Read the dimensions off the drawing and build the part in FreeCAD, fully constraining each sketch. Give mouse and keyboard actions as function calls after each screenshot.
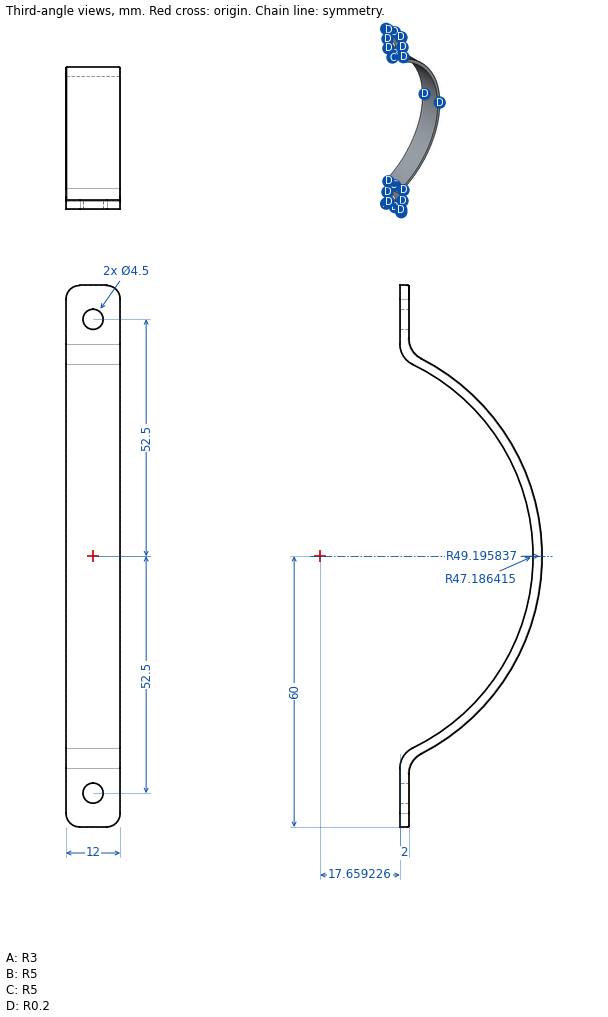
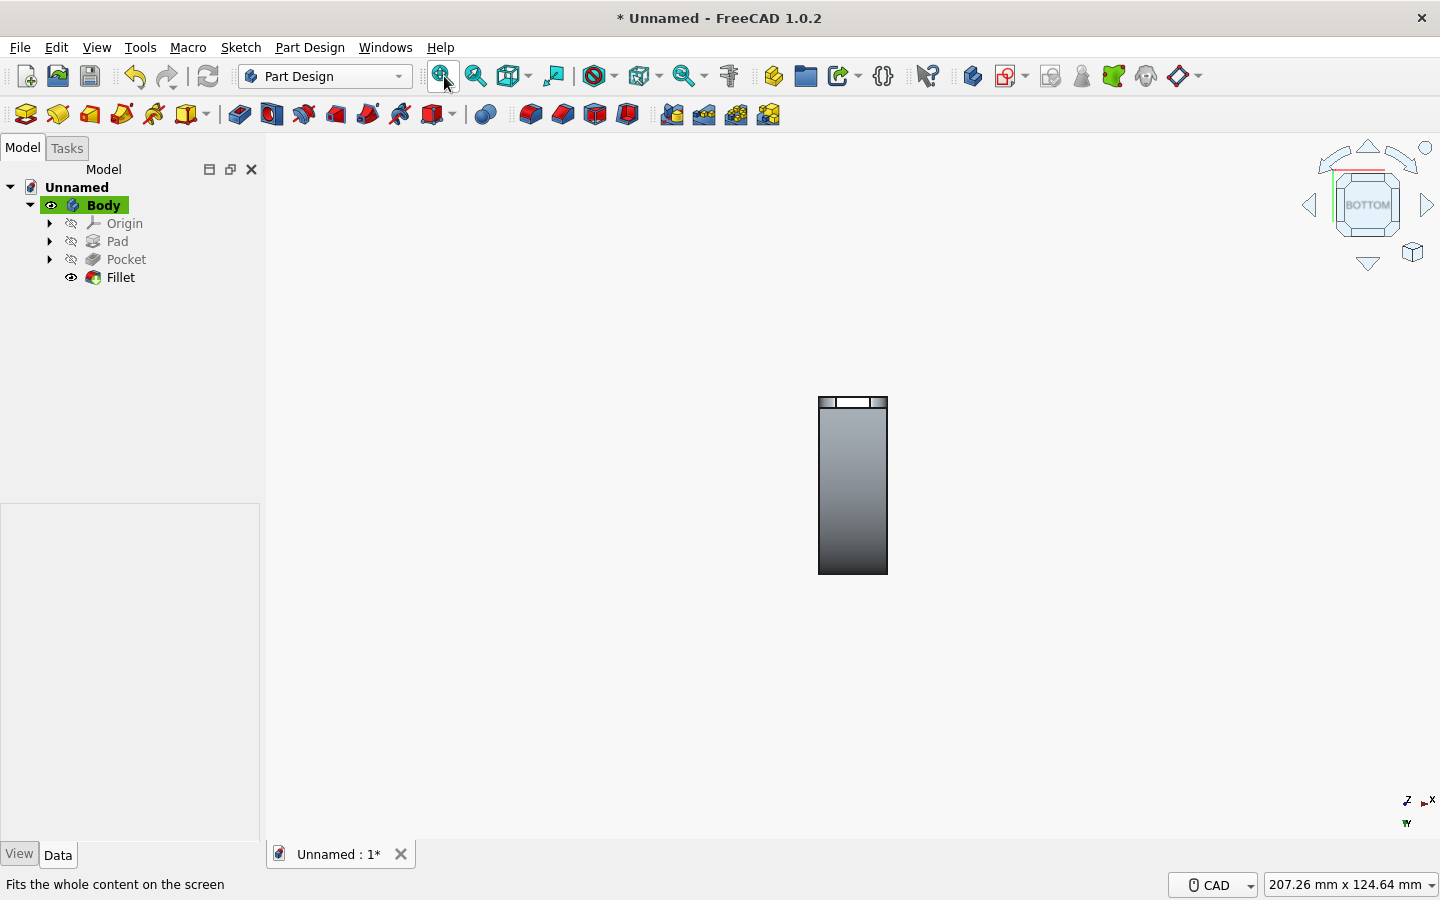
key(4)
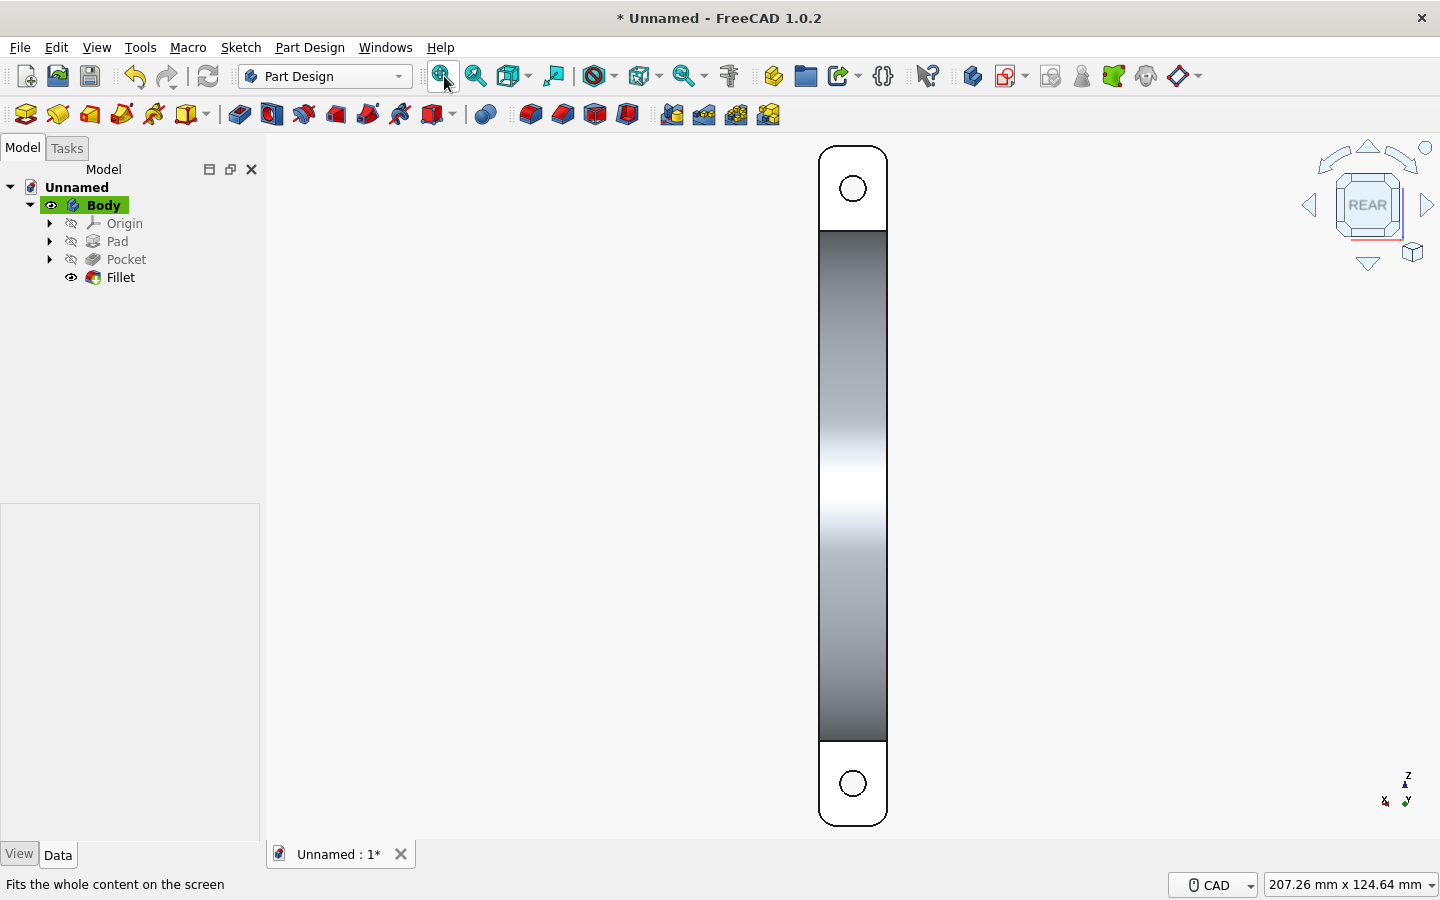
key(6)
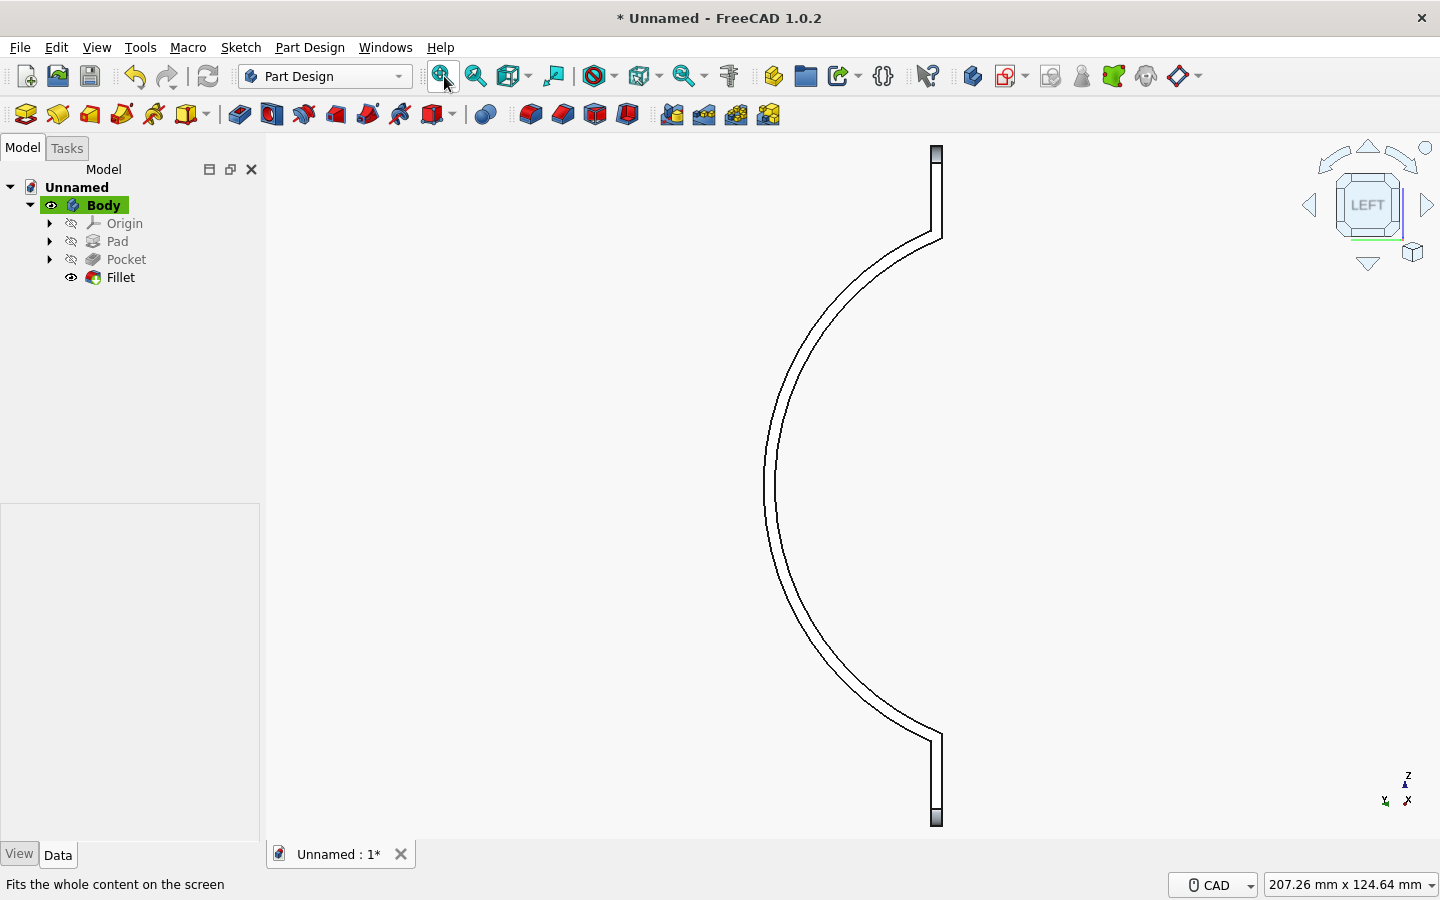
key(v)
key(3)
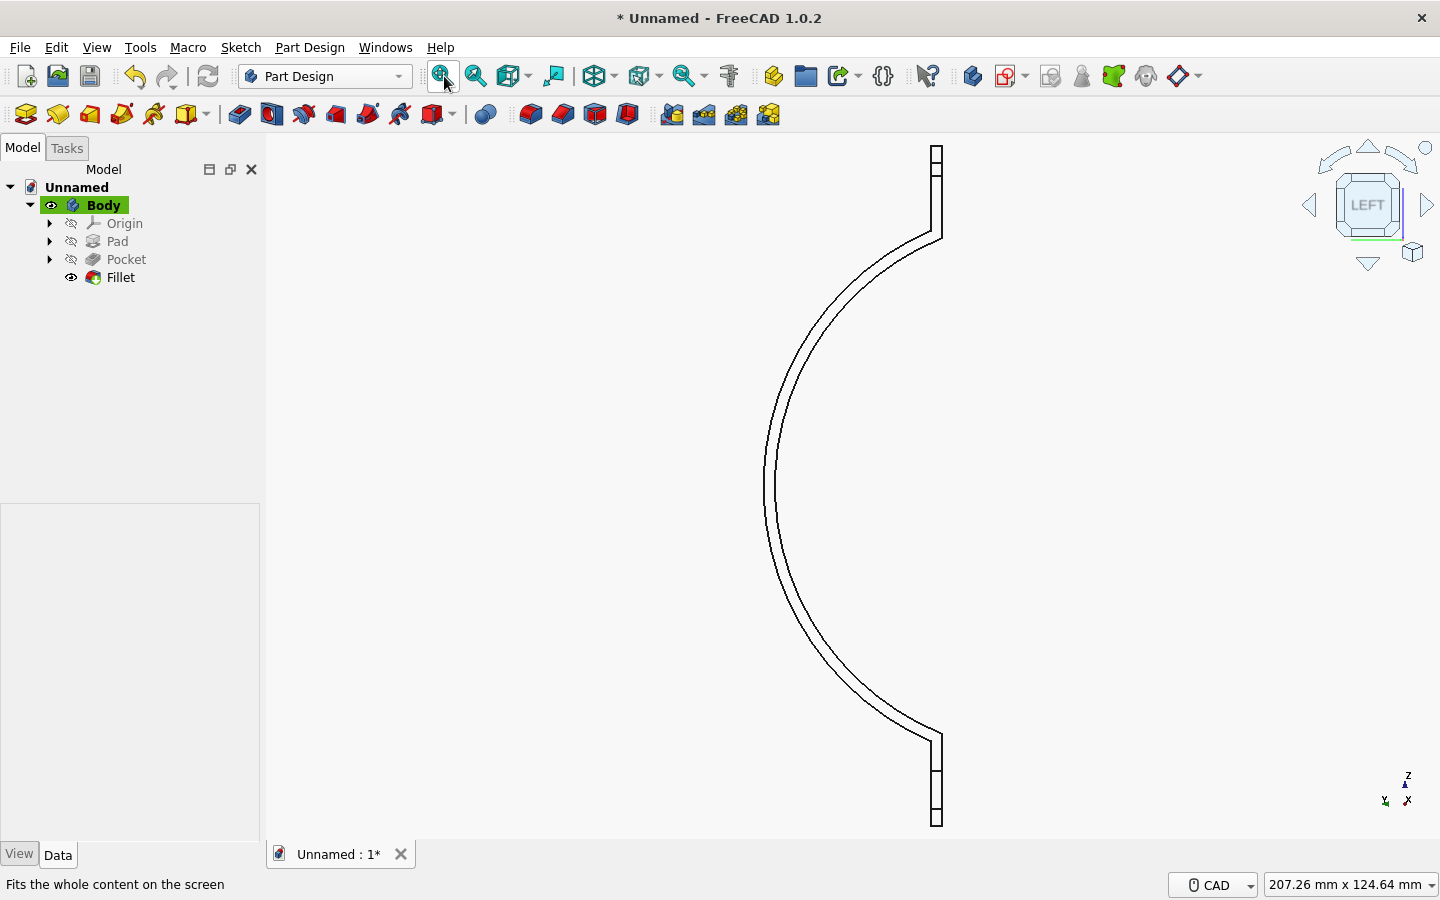
key(0)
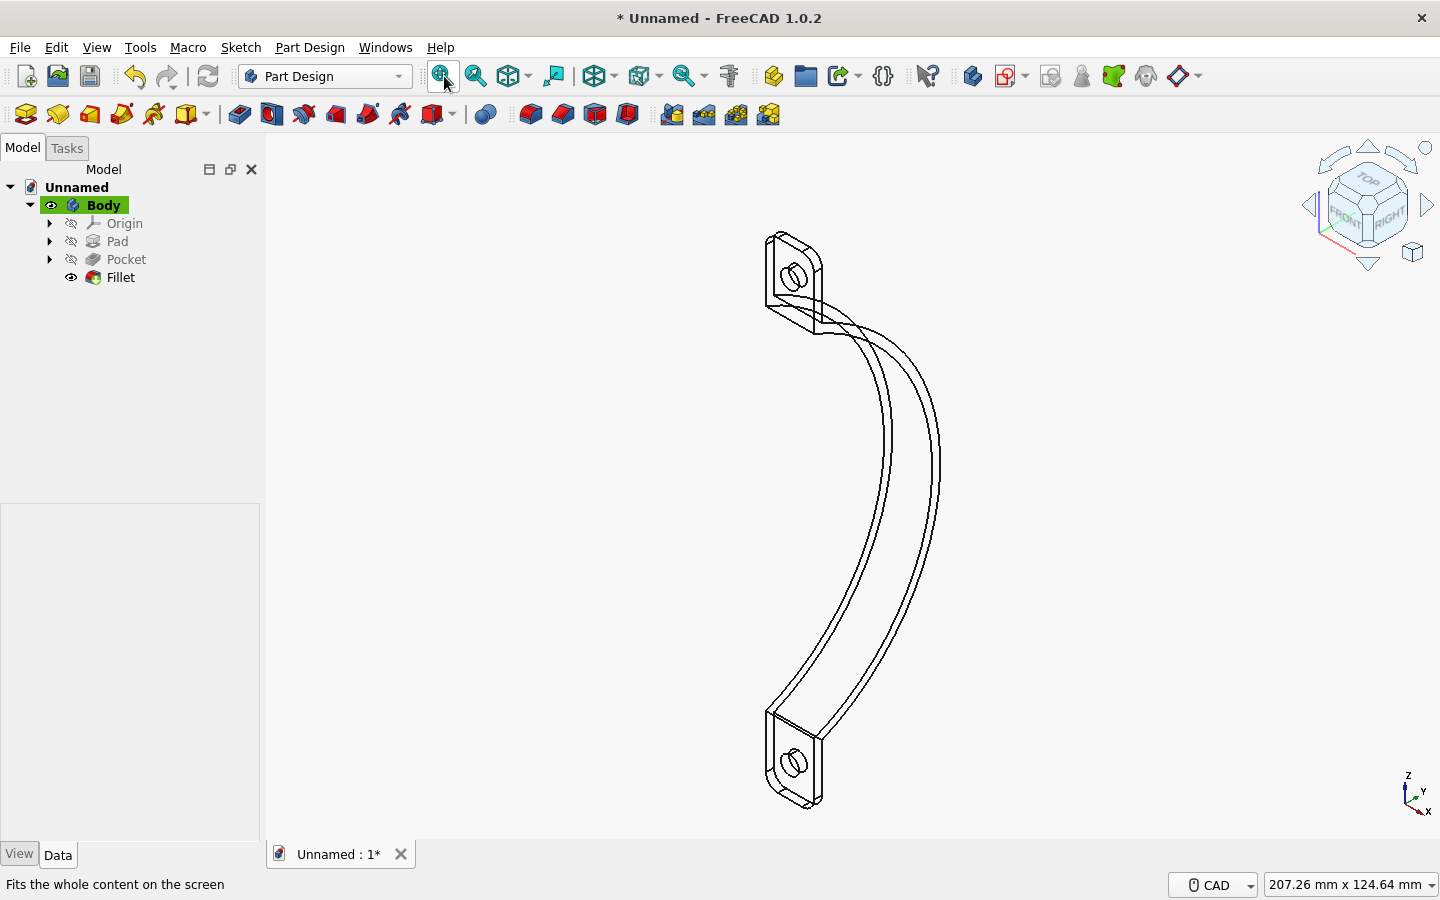
click(798, 308)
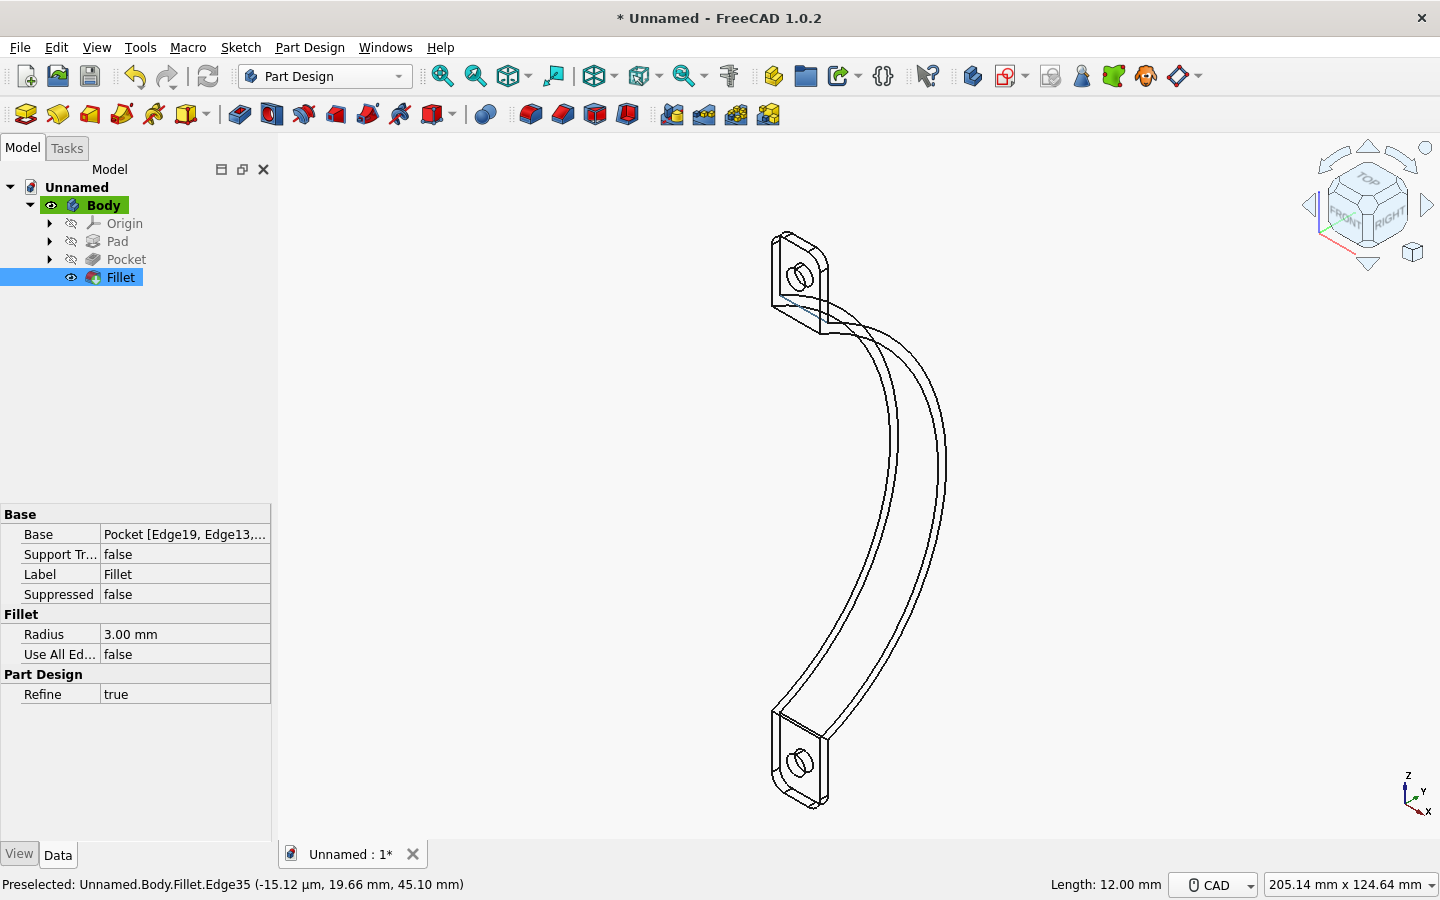
key(2)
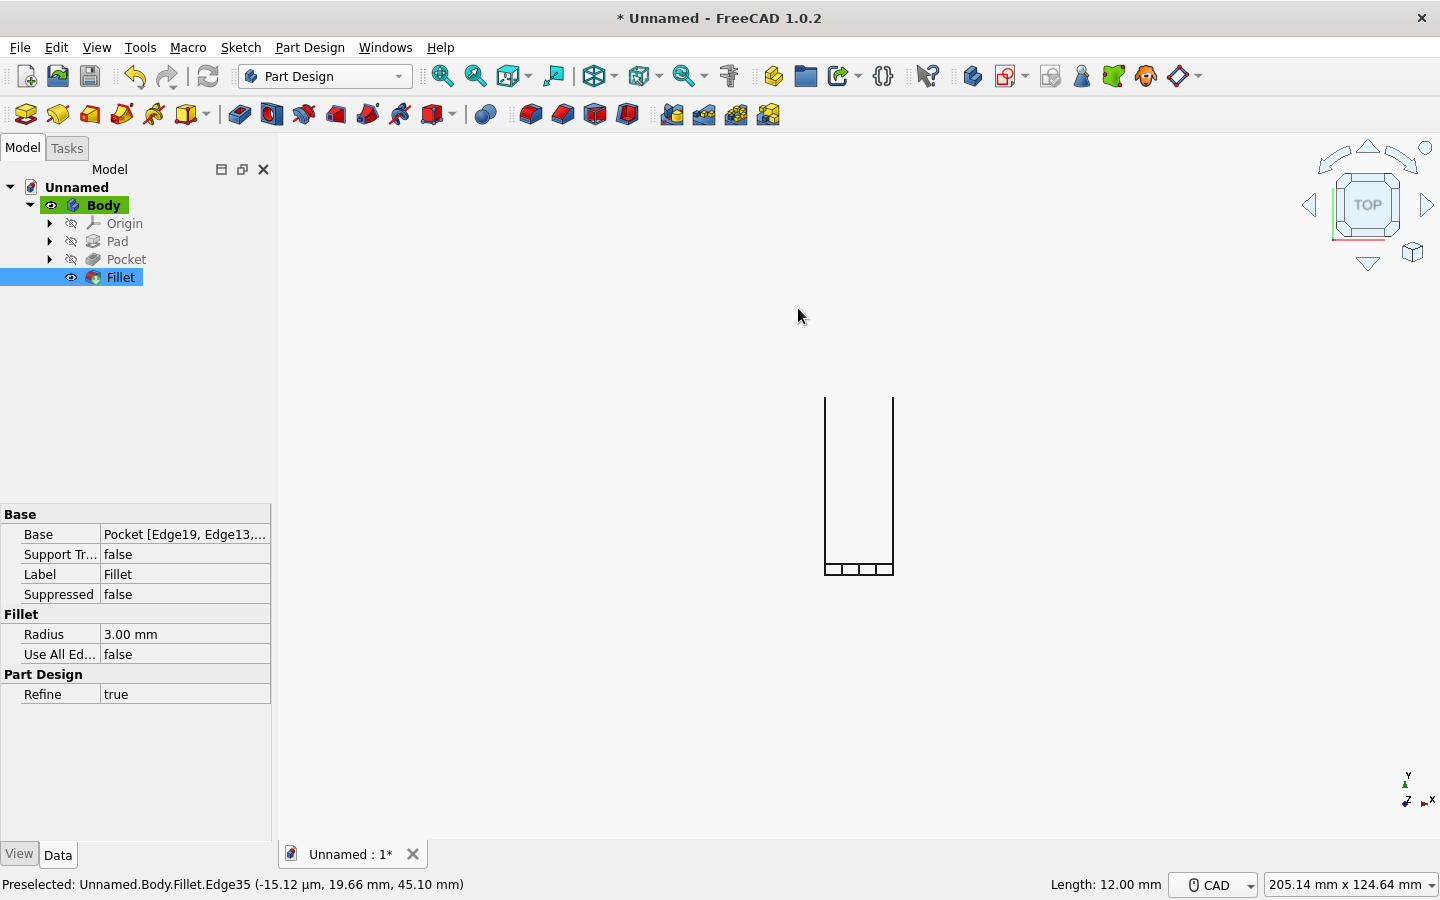
click(444, 76)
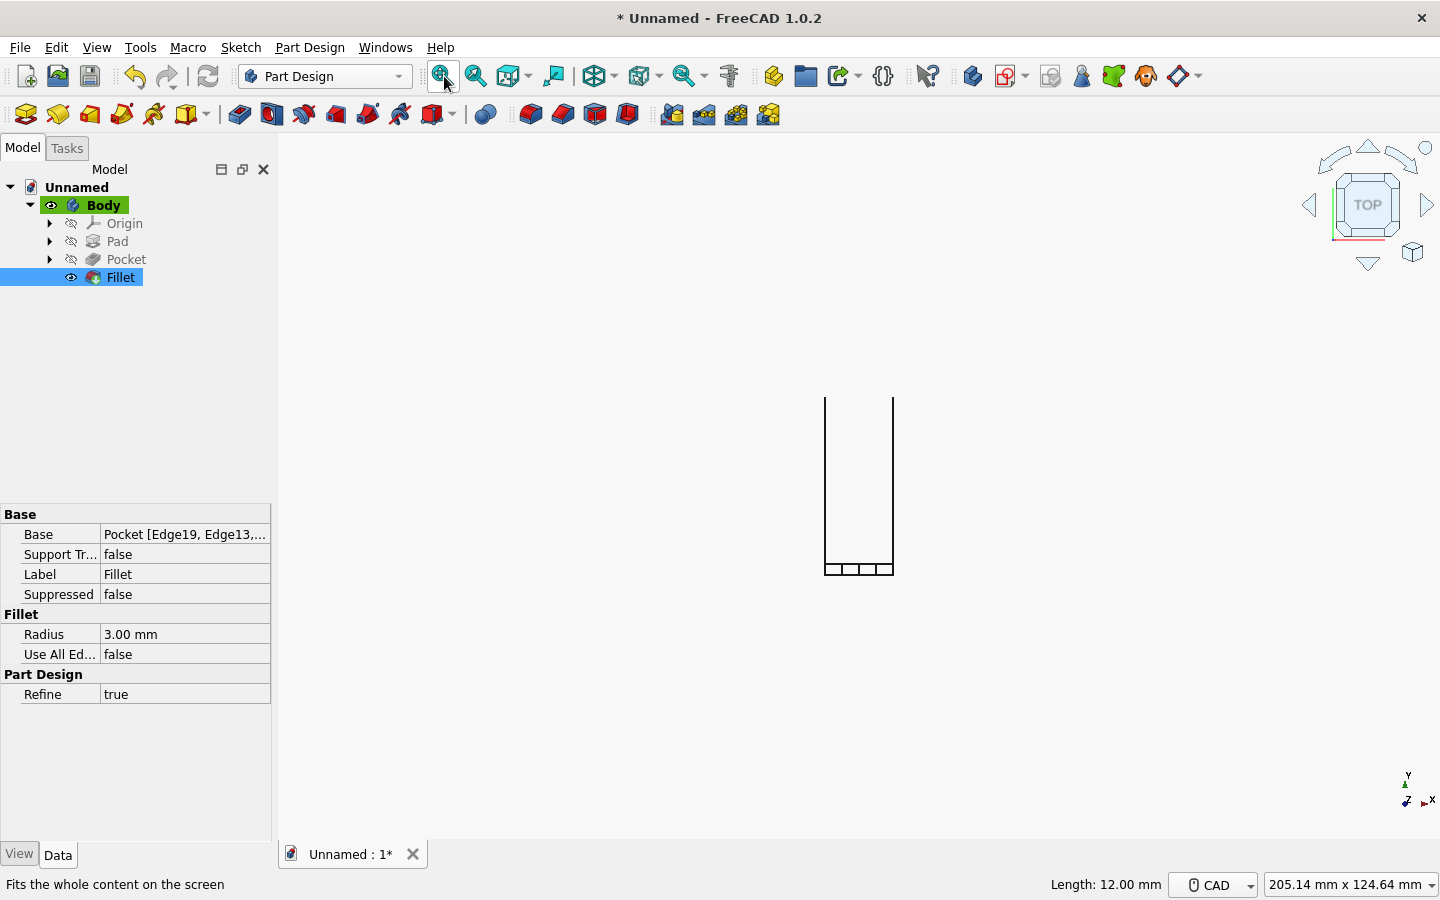
key(1)